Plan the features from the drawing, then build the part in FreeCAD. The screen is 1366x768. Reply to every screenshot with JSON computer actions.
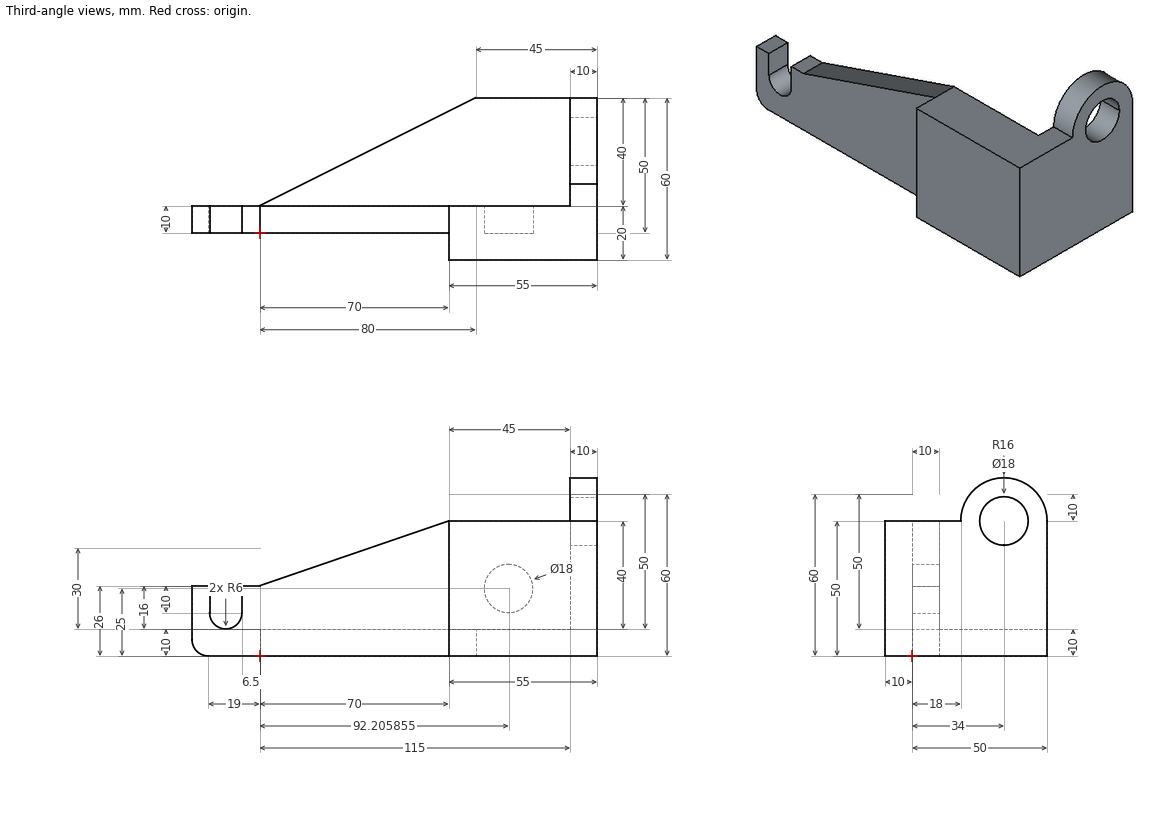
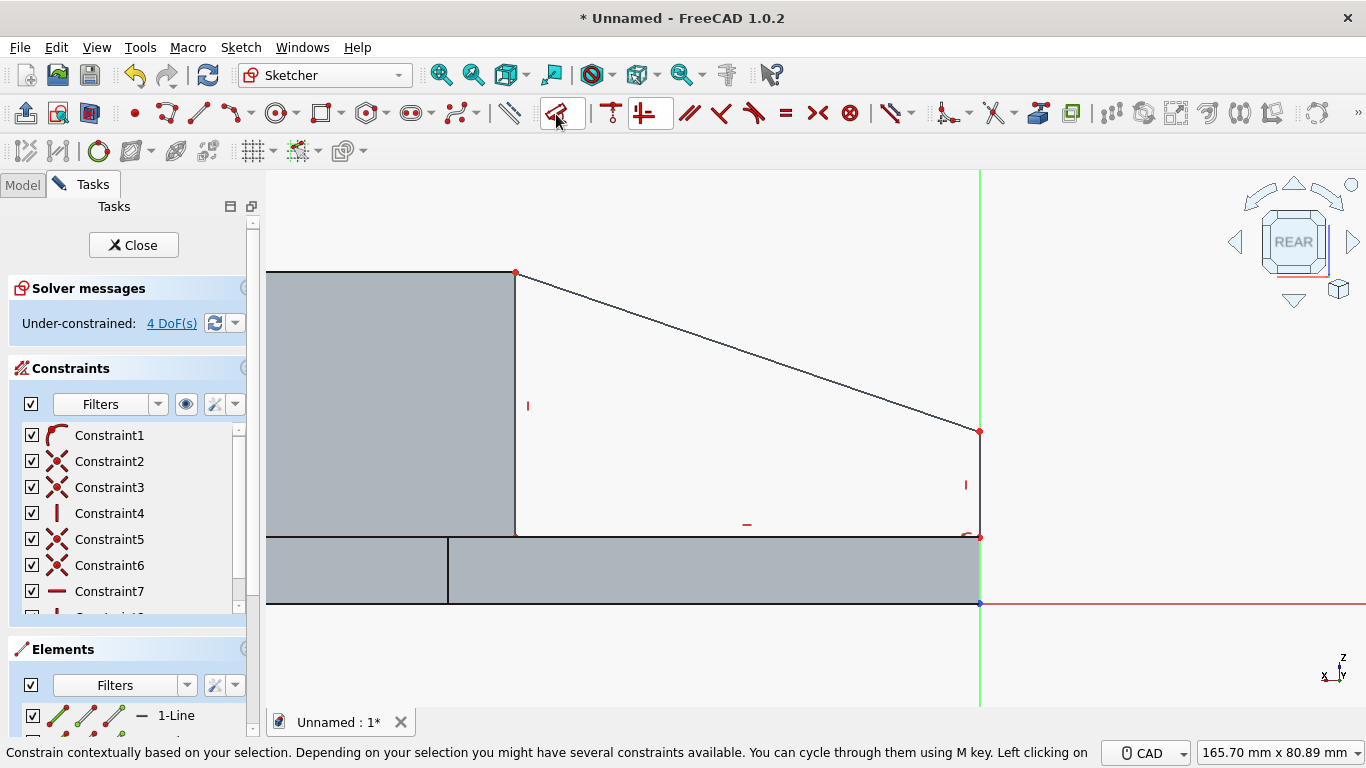
{"action": "left_click", "coordinate": [980, 506]}
{"action": "left_click", "coordinate": [1014, 485]}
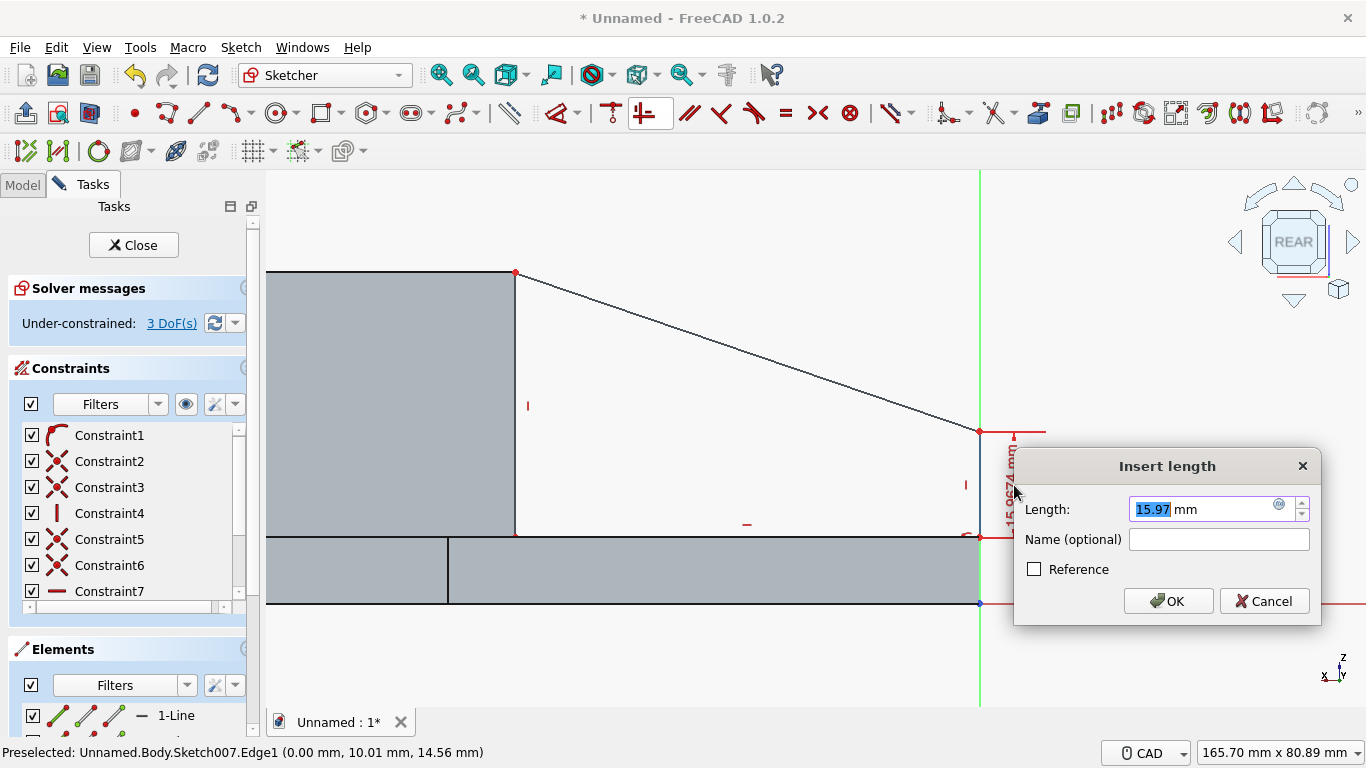
{"action": "type", "text": "16"}
{"action": "key", "text": "Return"}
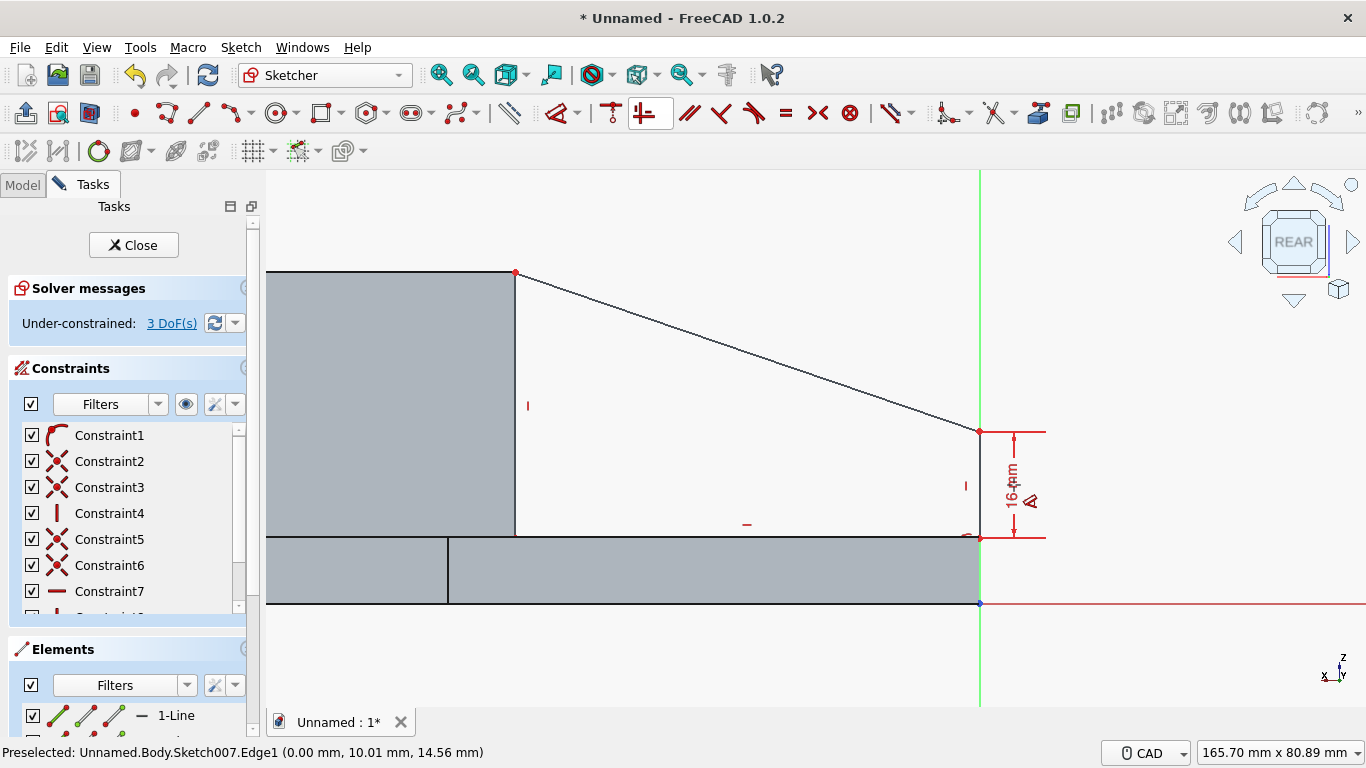
{"action": "left_click", "coordinate": [515, 353]}
{"action": "left_click", "coordinate": [481, 406]}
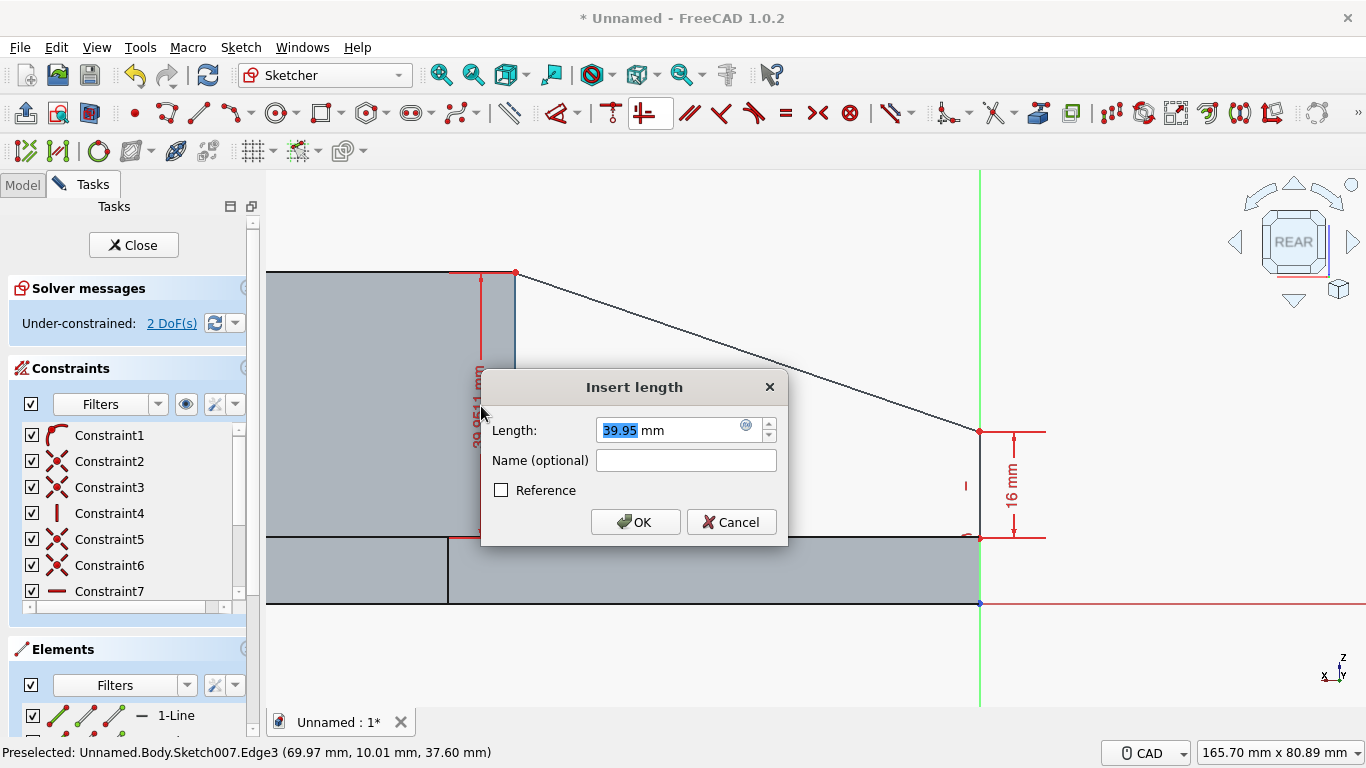
{"action": "type", "text": "40"}
{"action": "key", "text": "Return"}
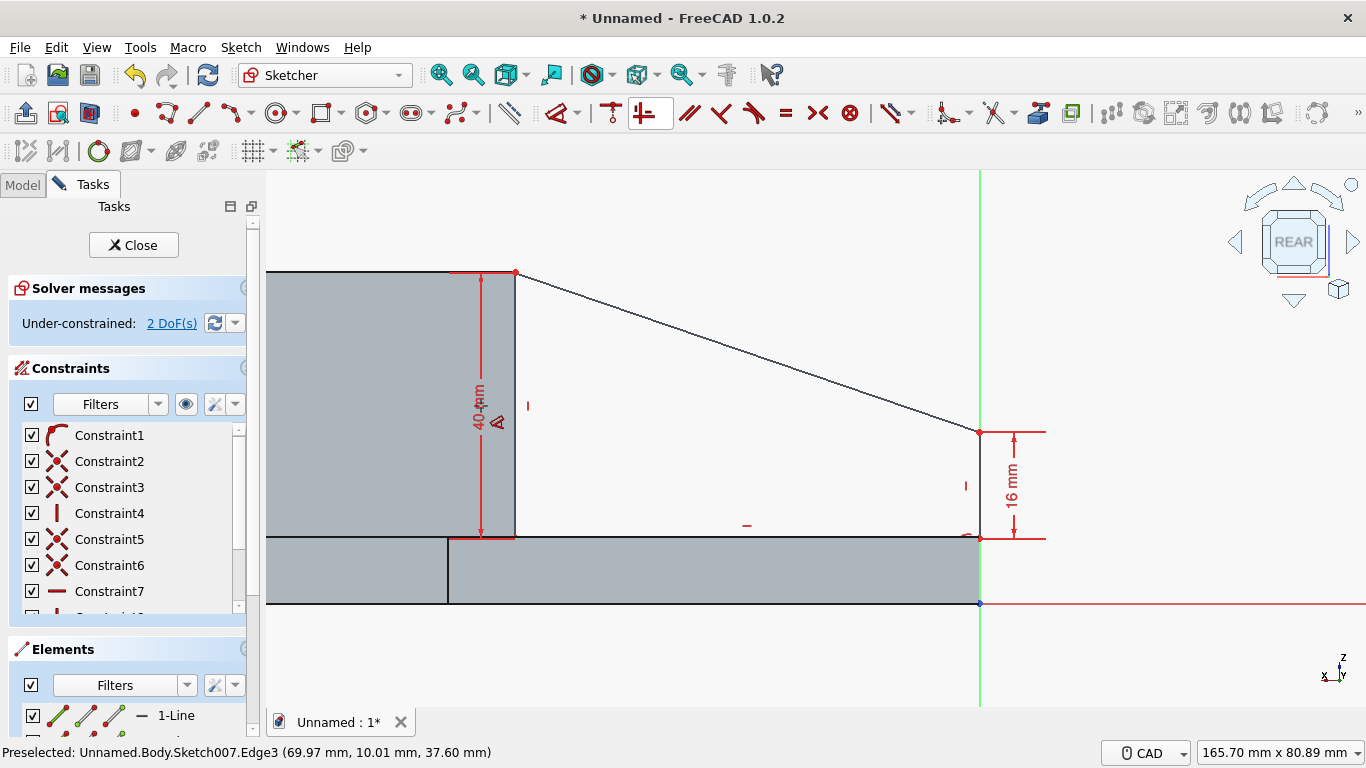
{"action": "left_click", "coordinate": [654, 539]}
{"action": "left_click", "coordinate": [747, 573]}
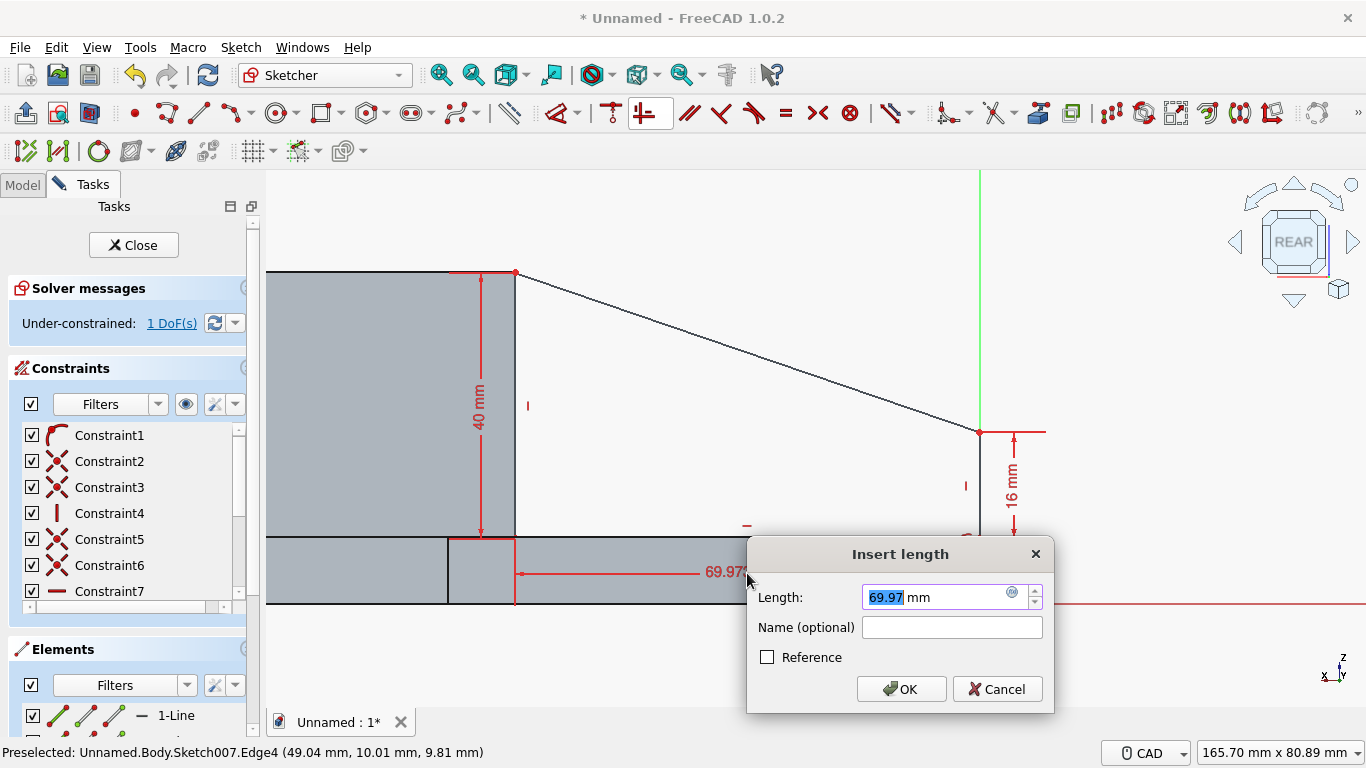
{"action": "type", "text": "70"}
{"action": "key", "text": "Return"}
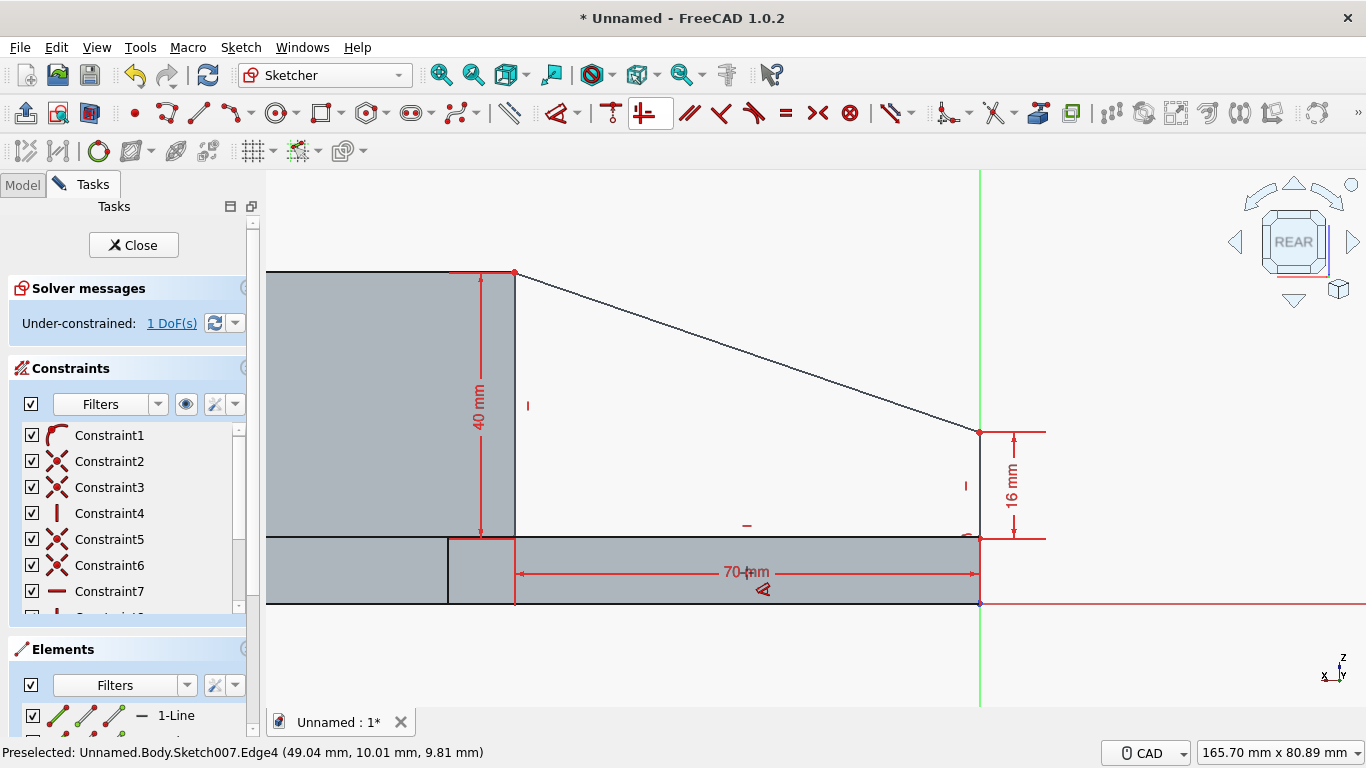
{"action": "left_click", "coordinate": [980, 539]}
{"action": "left_click", "coordinate": [1014, 571]}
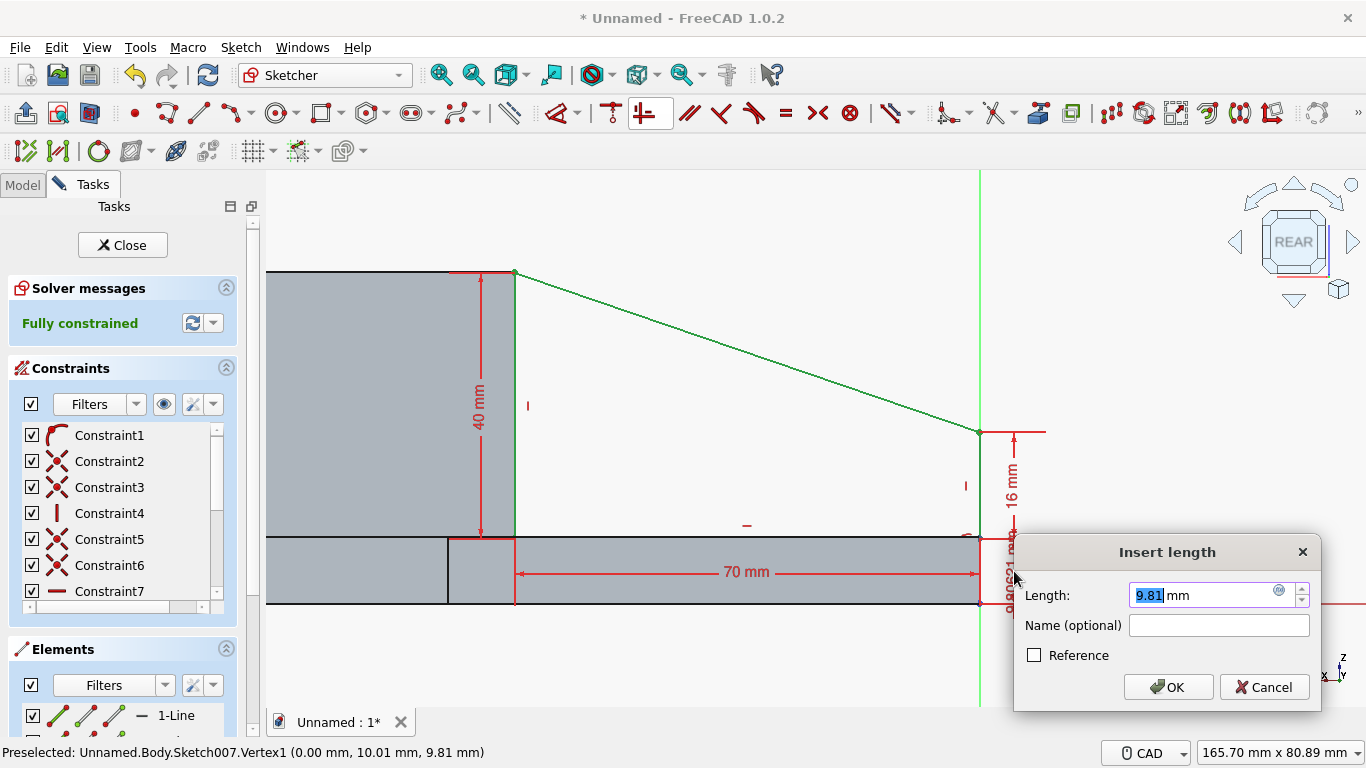
{"action": "type", "text": "10"}
{"action": "key", "text": "Return"}
{"action": "key", "text": "Escape"}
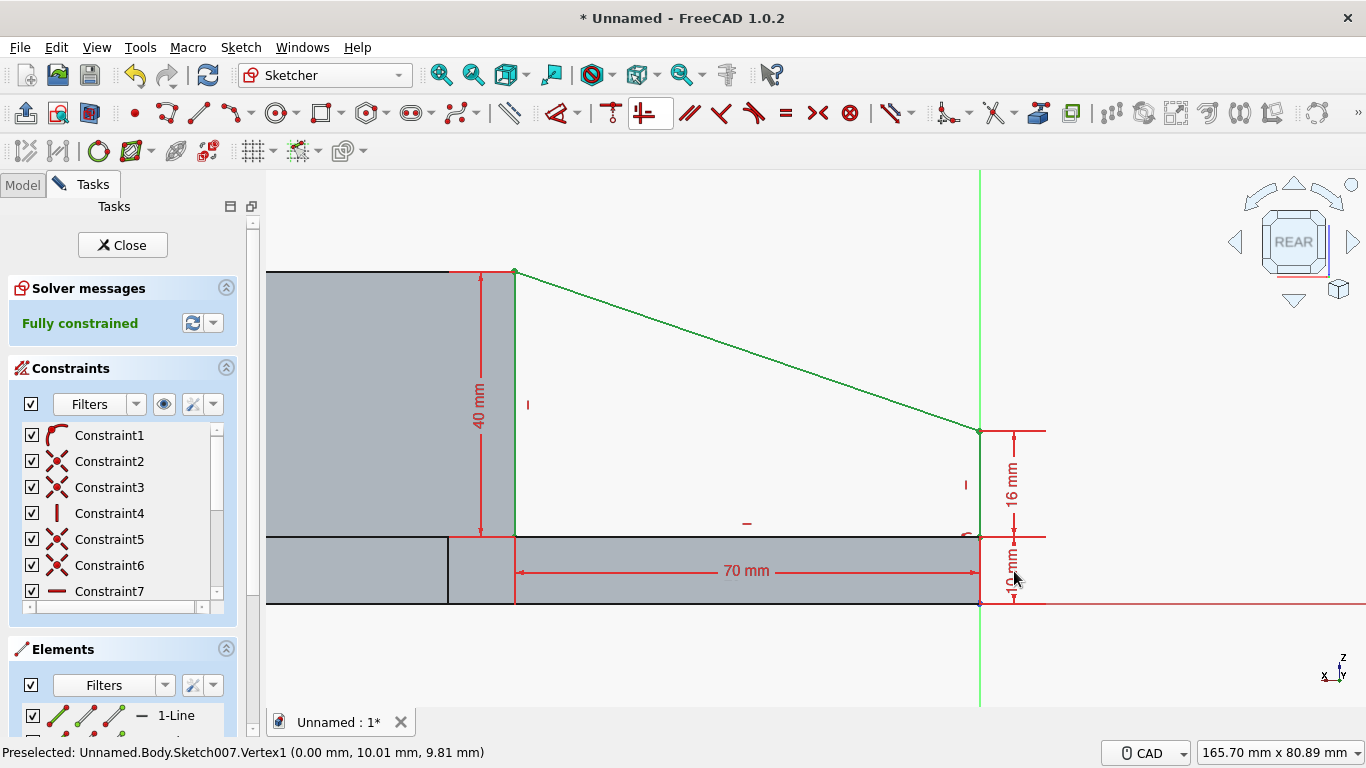
{"action": "left_click", "coordinate": [123, 245]}